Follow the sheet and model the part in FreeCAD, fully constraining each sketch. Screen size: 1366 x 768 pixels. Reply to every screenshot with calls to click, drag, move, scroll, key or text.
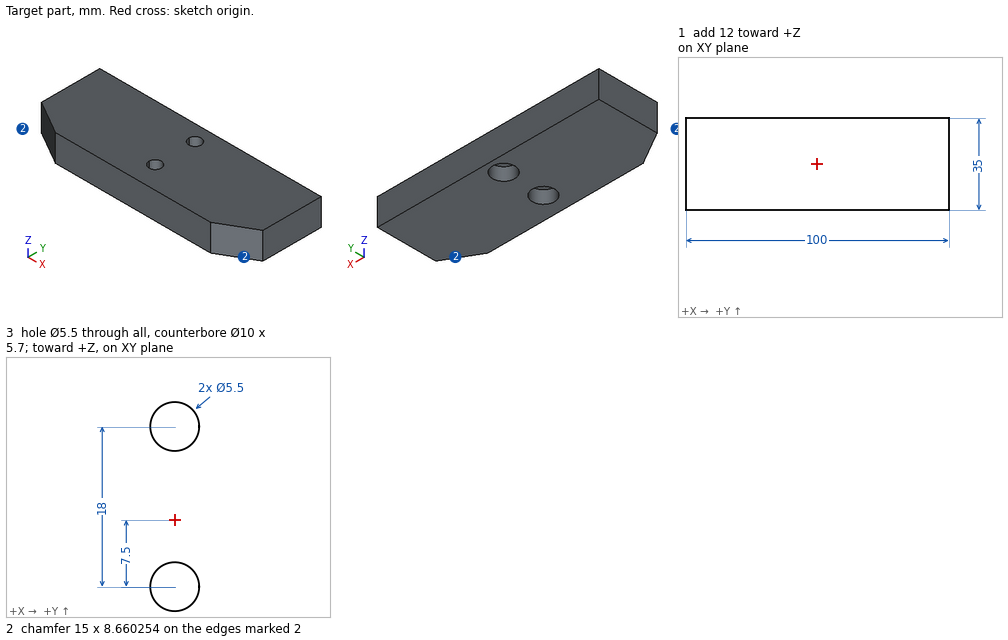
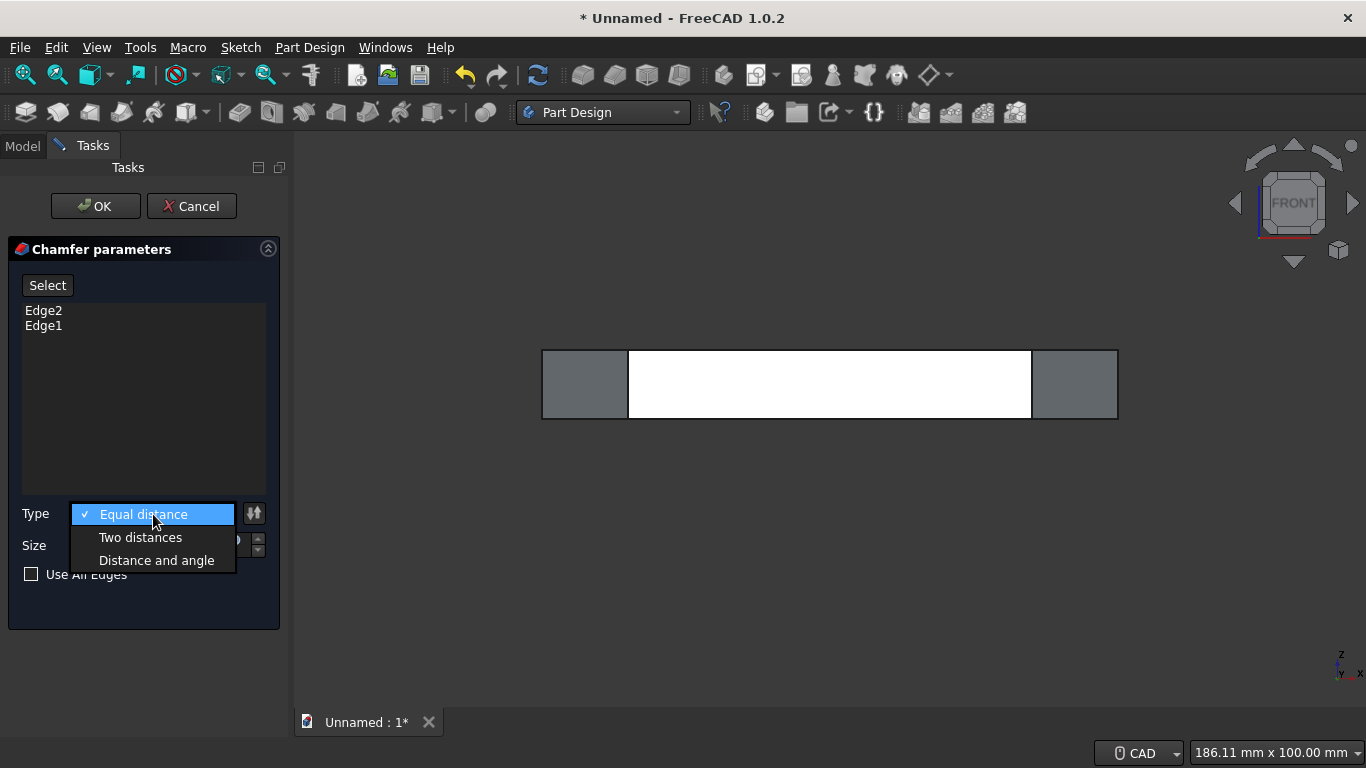
click(152, 538)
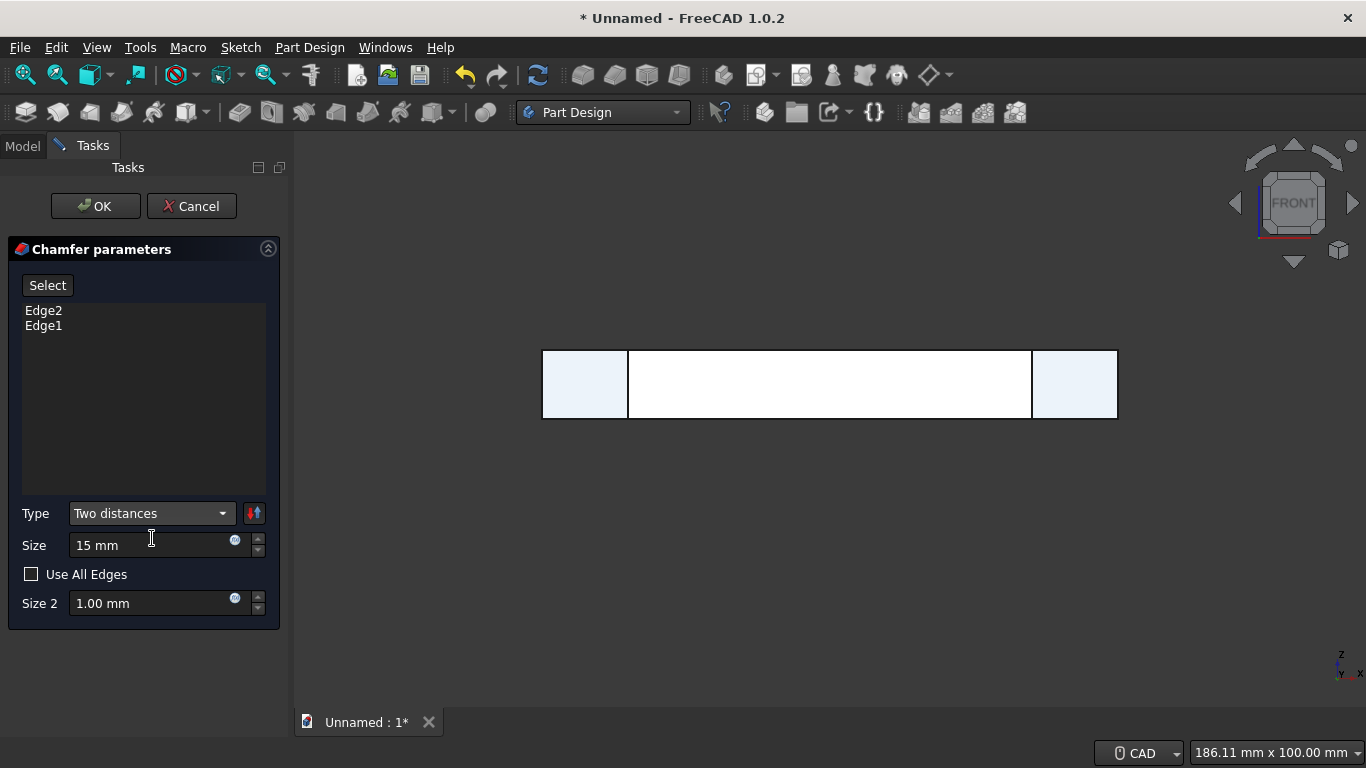
triple_click(160, 603)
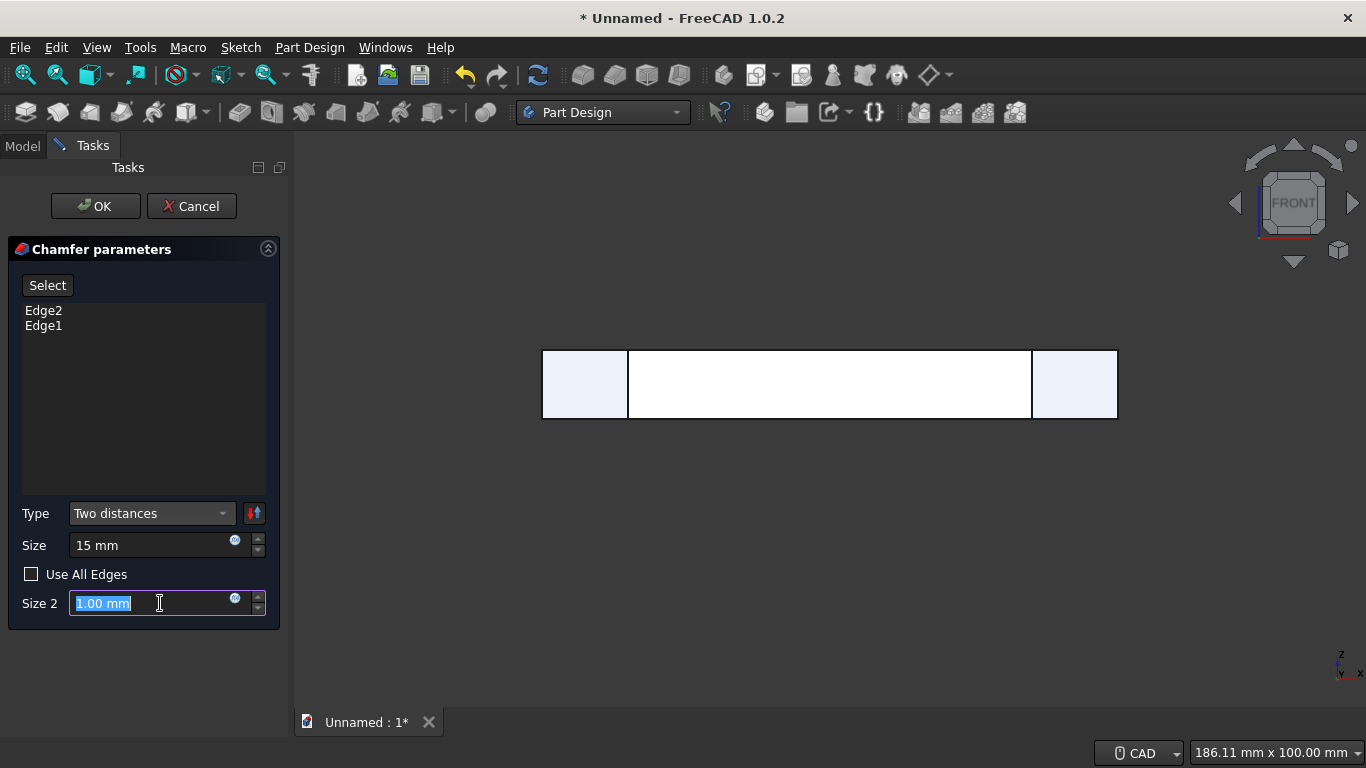
text(8.660254)
key(Tab)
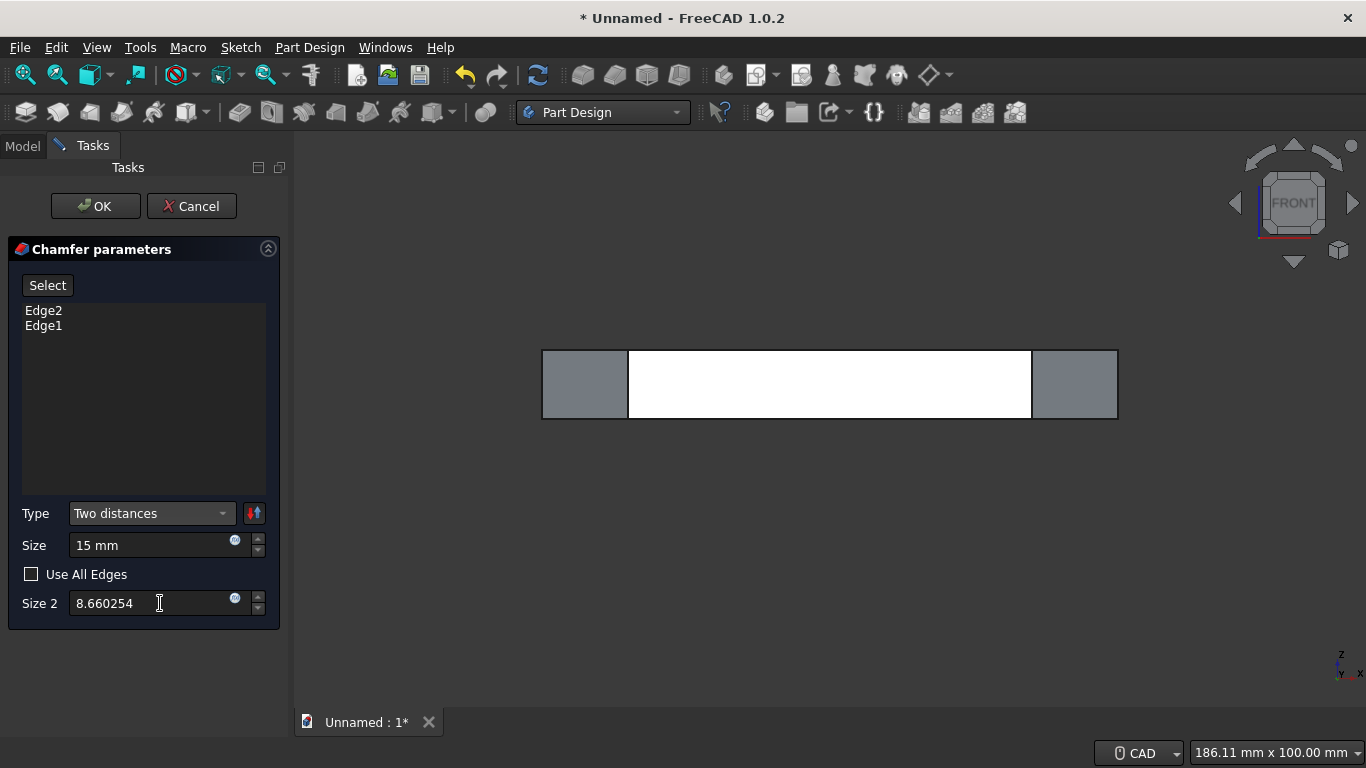
click(96, 206)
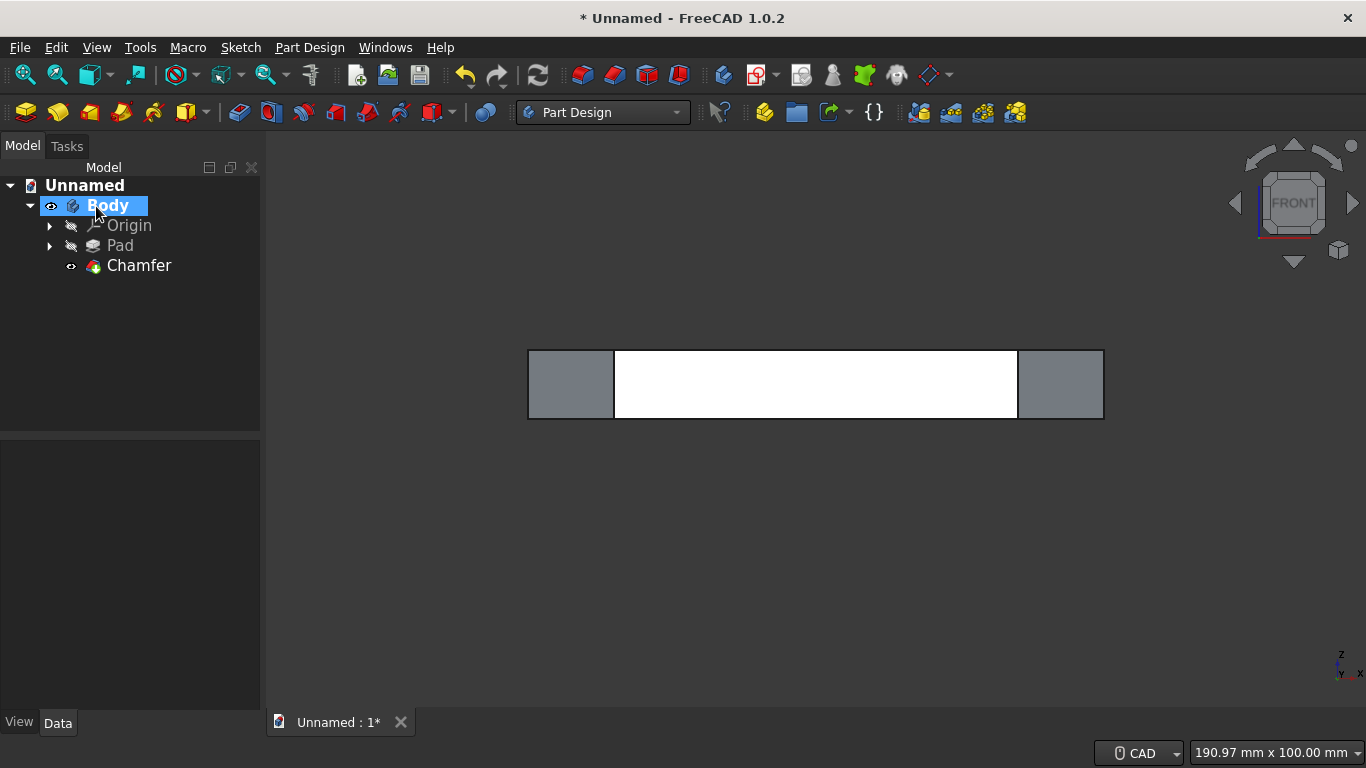
click(756, 76)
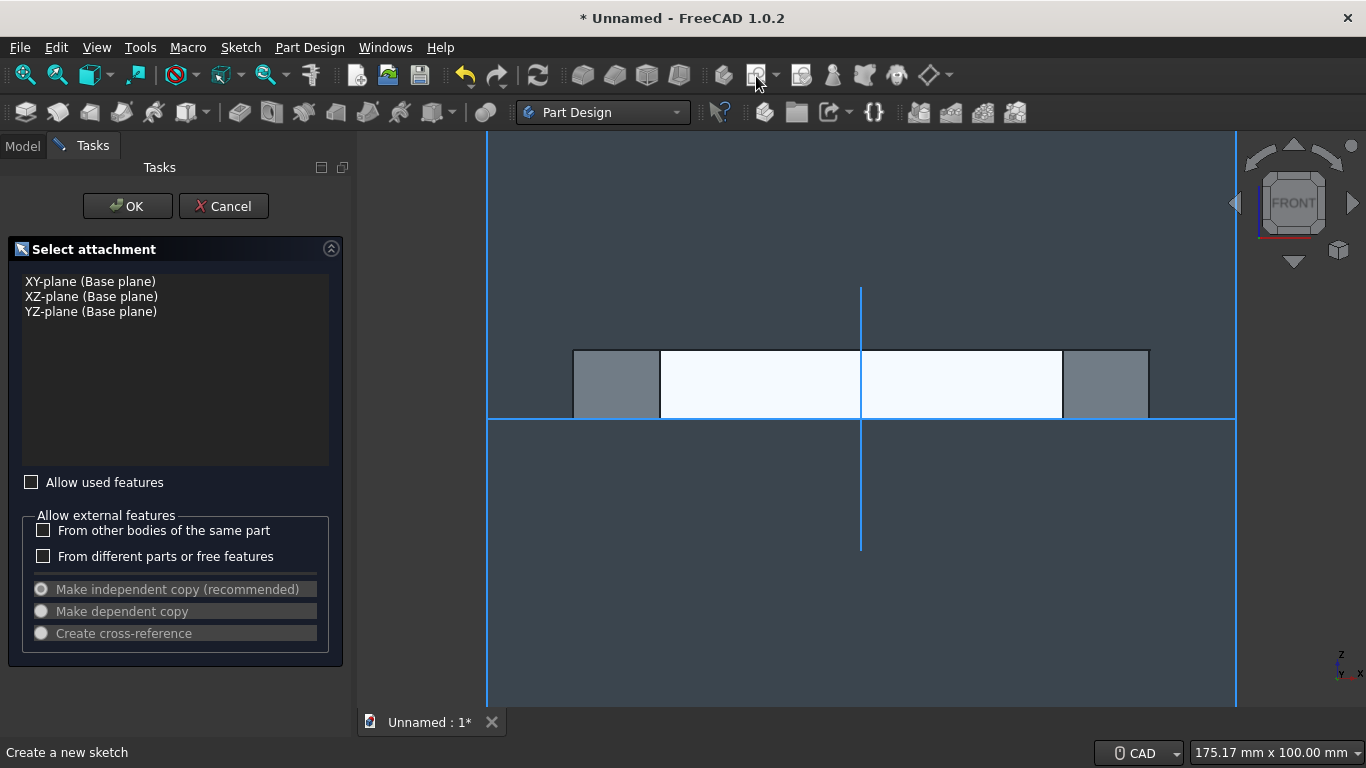
click(82, 282)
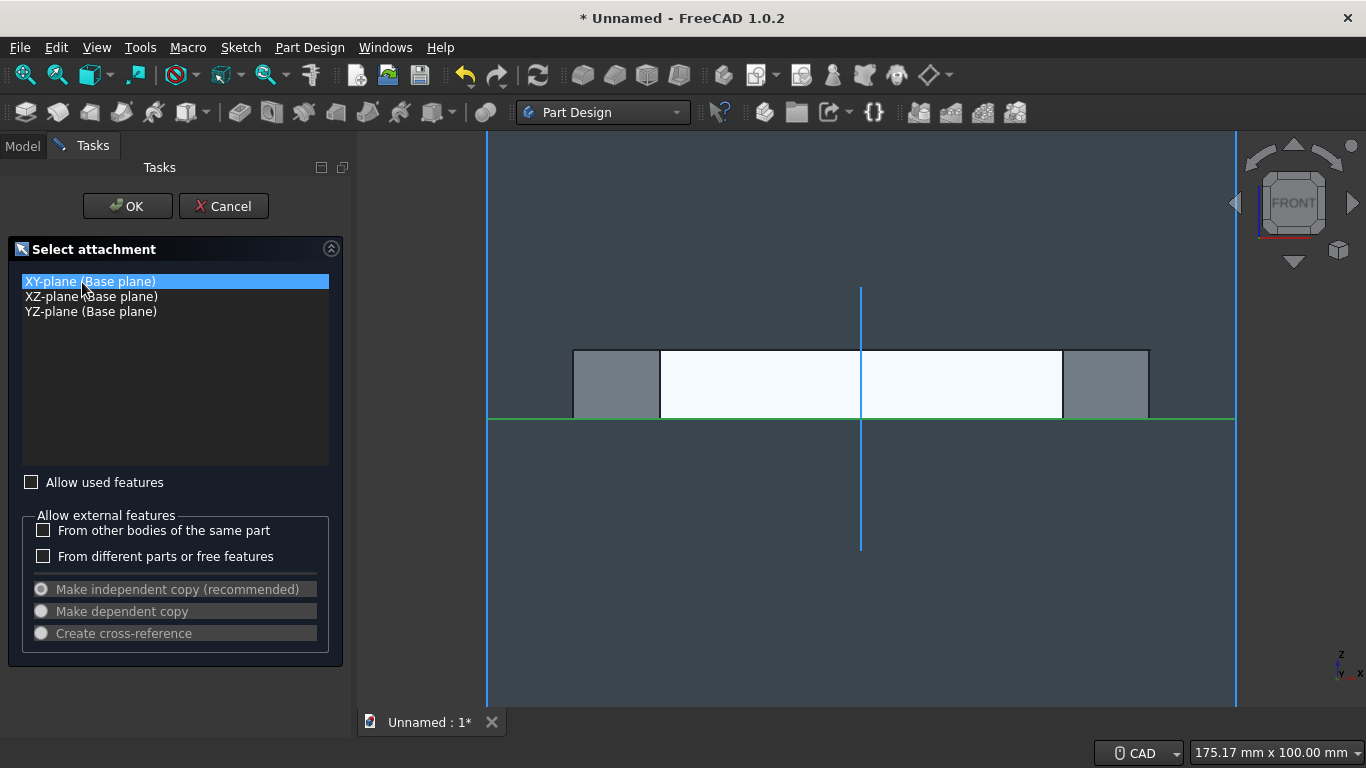
click(128, 206)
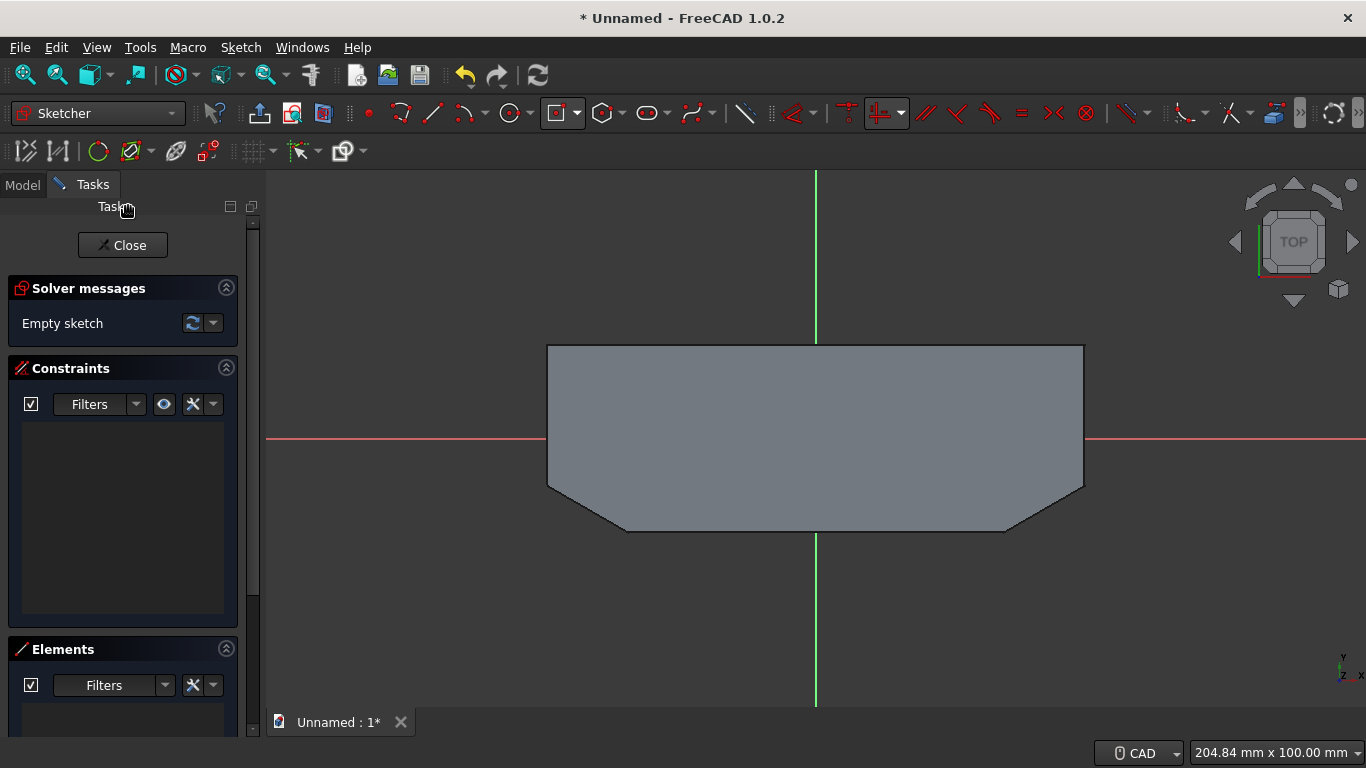
click(324, 114)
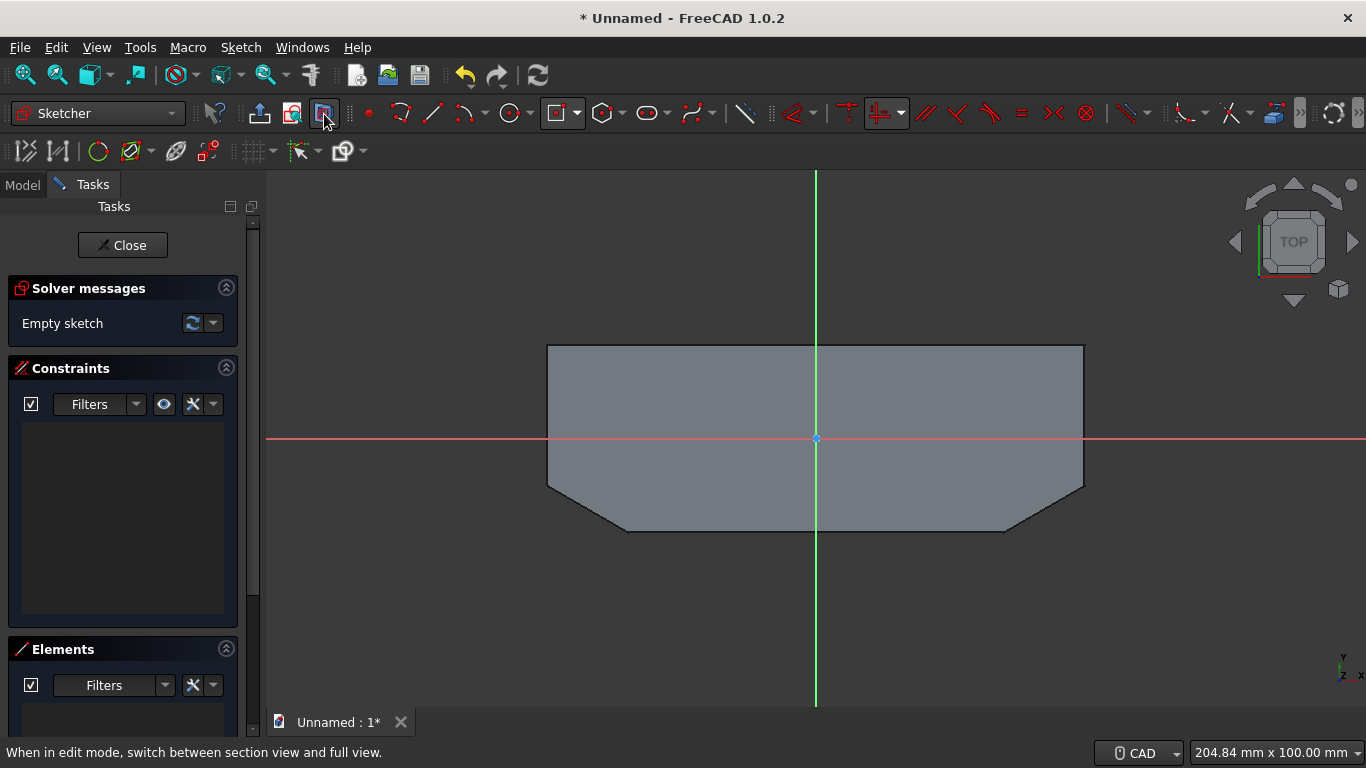
scroll(856, 426, up, 5)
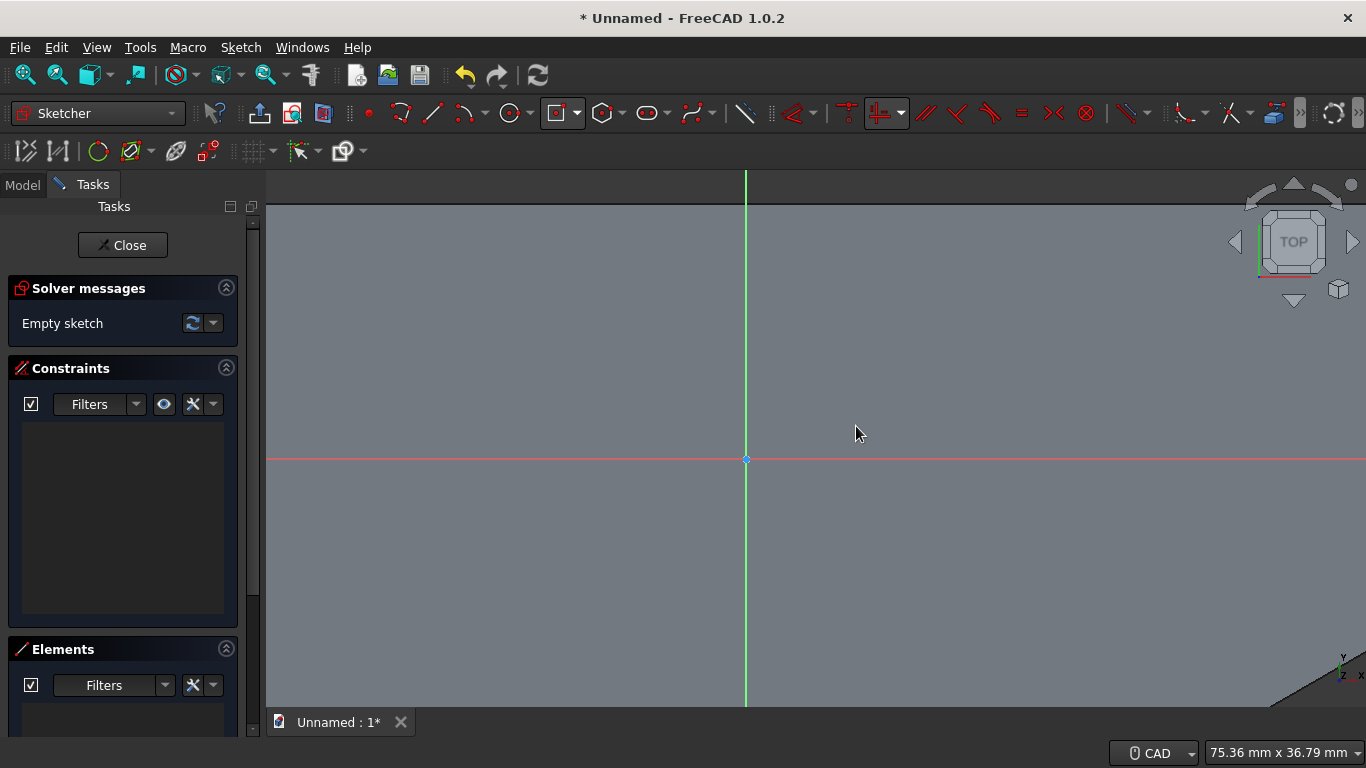
click(510, 114)